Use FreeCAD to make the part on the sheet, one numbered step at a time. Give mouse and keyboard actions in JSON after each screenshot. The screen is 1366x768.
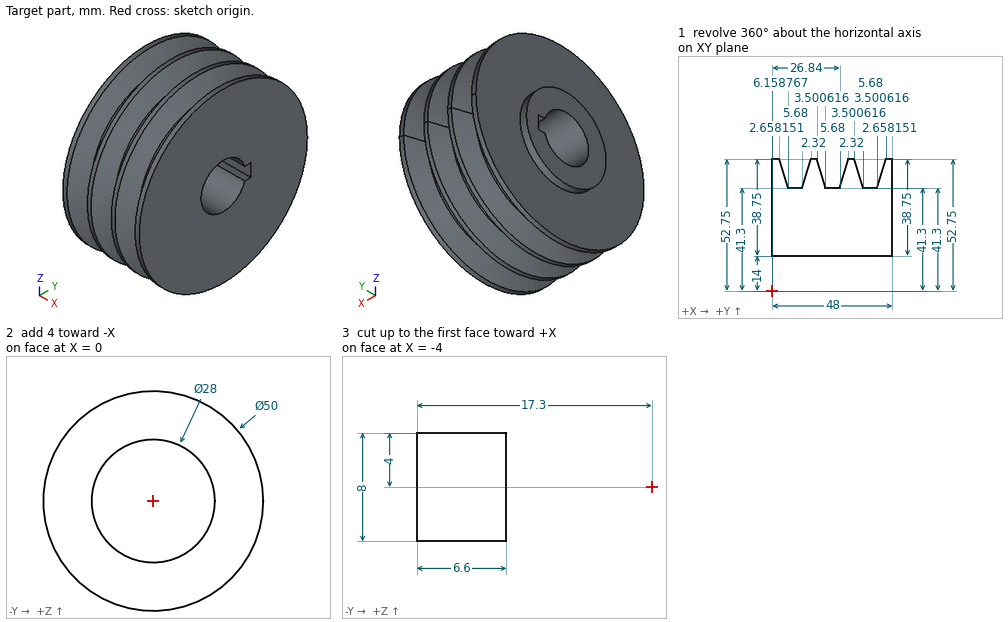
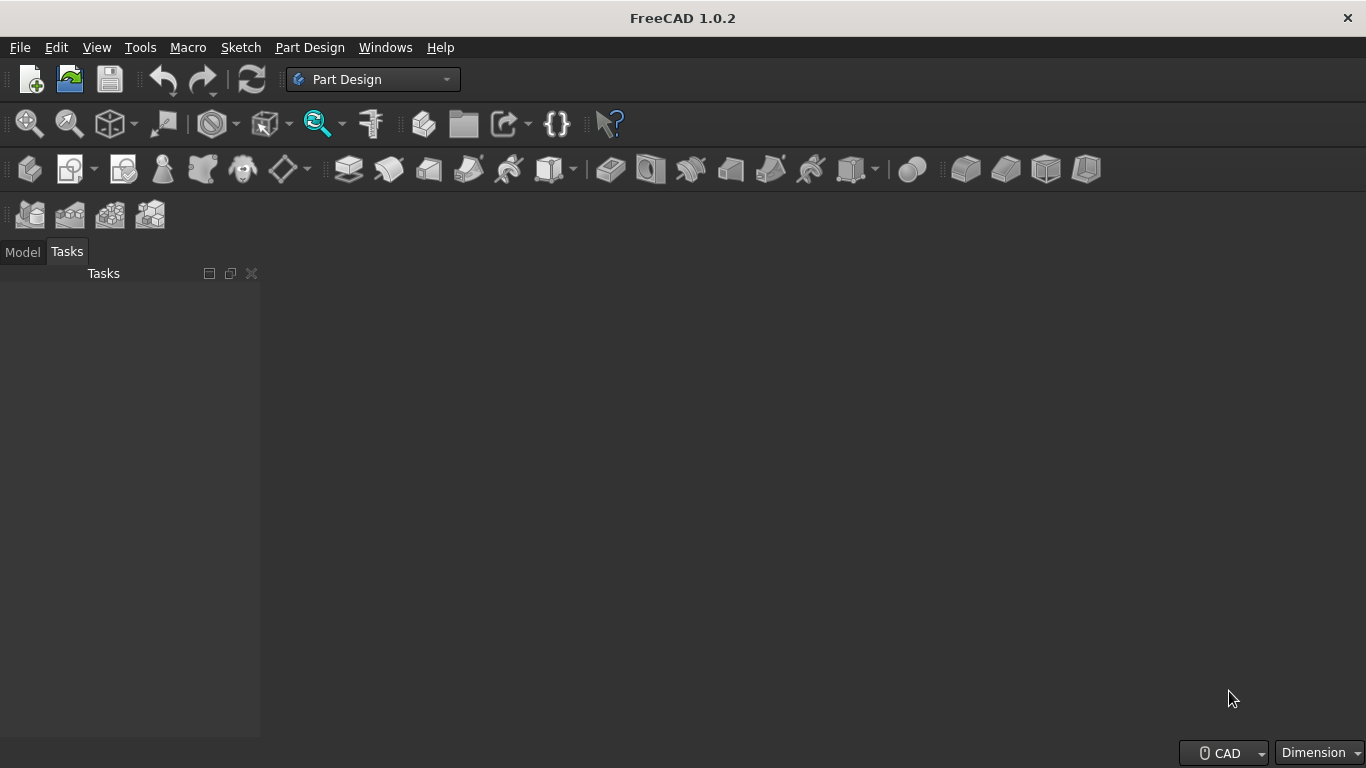
{"action": "left_click", "coordinate": [30, 80]}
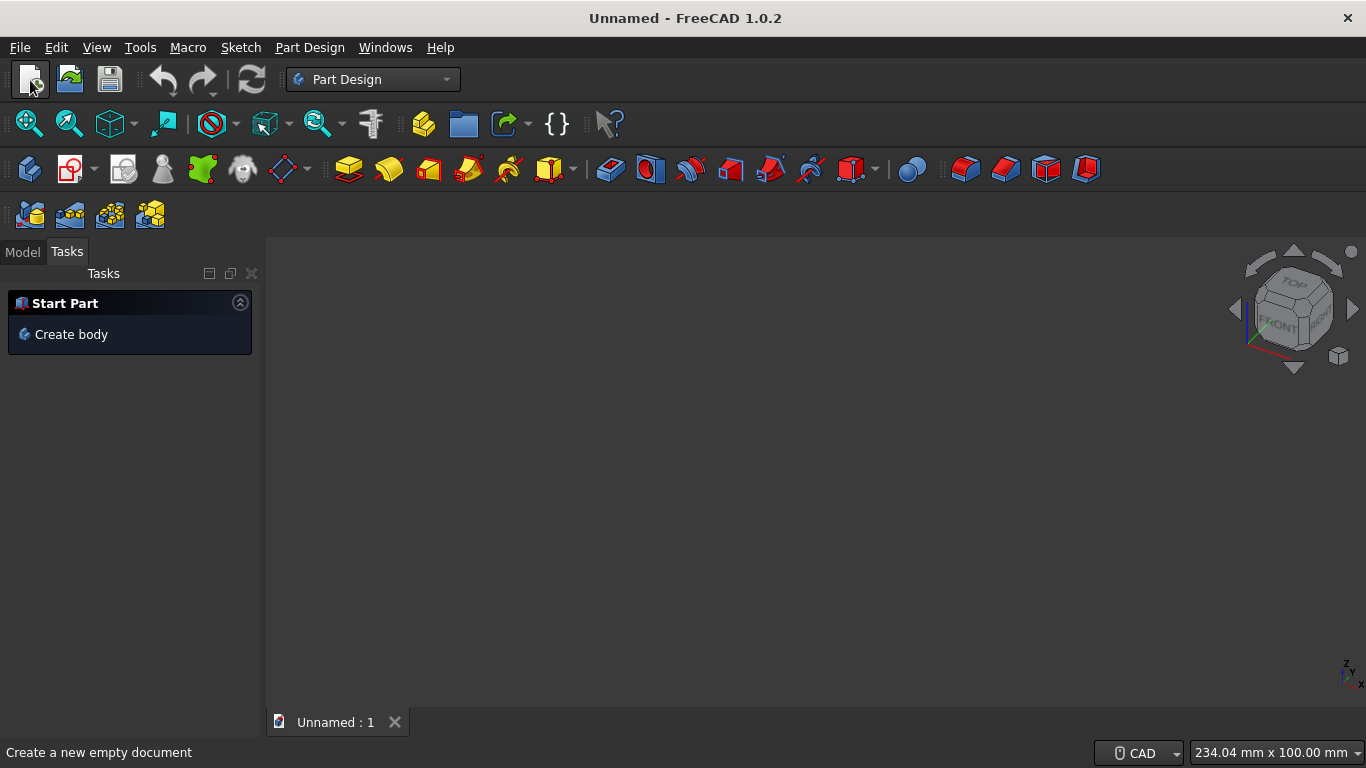
{"action": "left_click", "coordinate": [70, 170]}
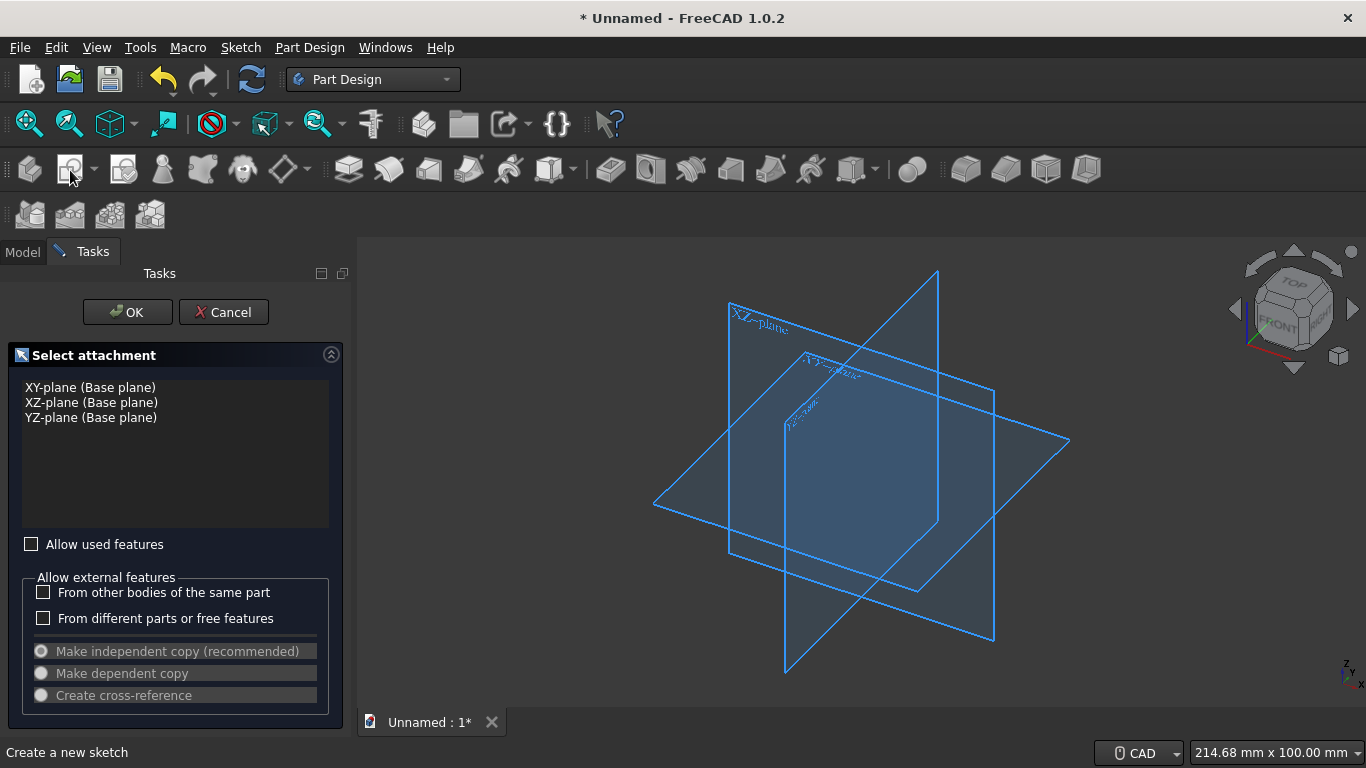
{"action": "left_click", "coordinate": [82, 388]}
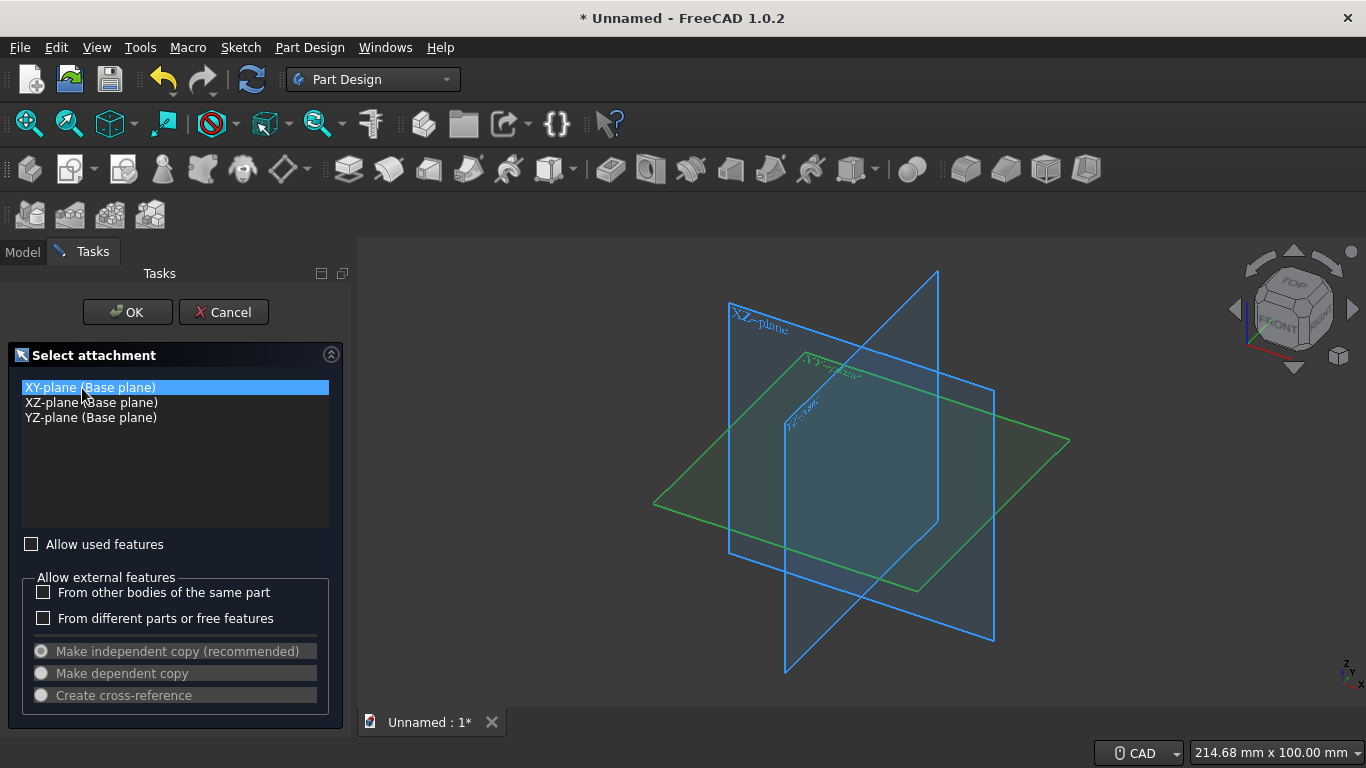
{"action": "left_click", "coordinate": [128, 312]}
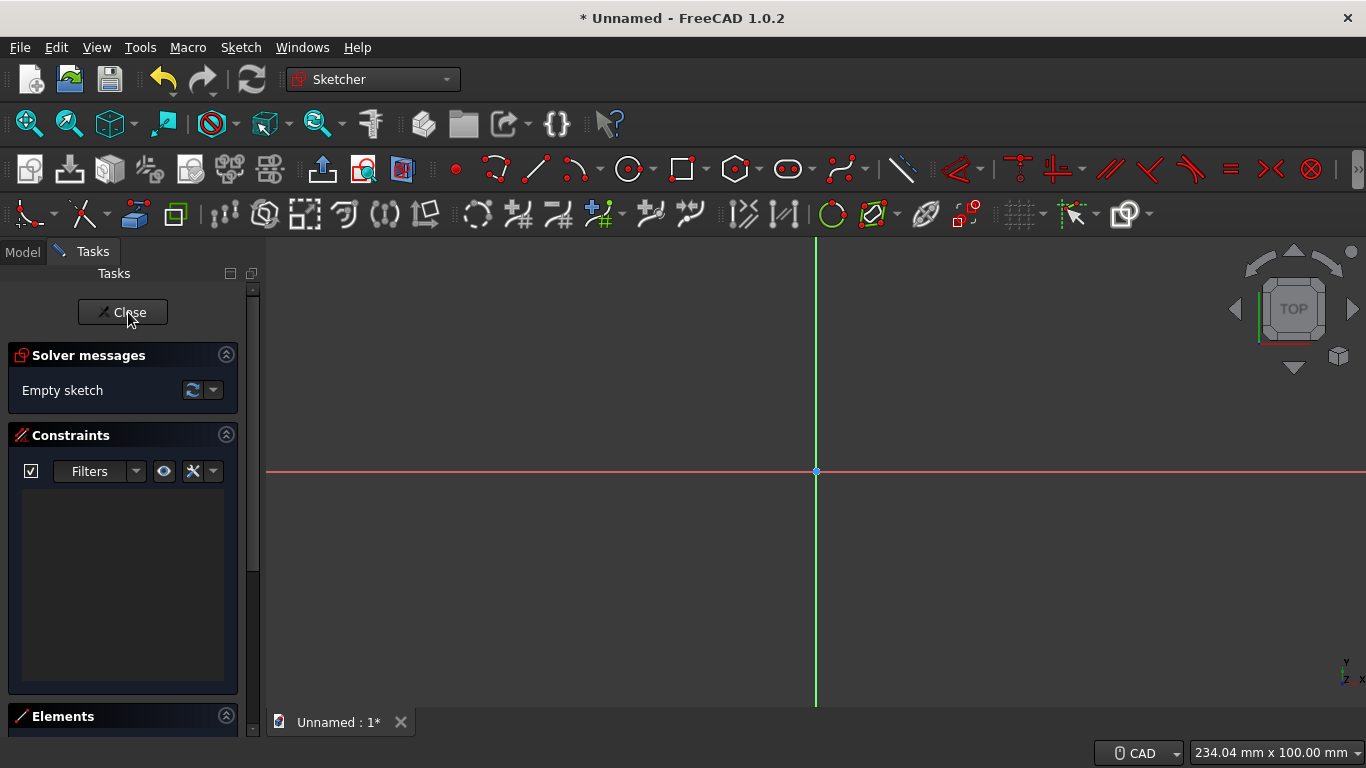
{"action": "scroll", "coordinate": [294, 679], "scroll_direction": "down", "scroll_amount": 1}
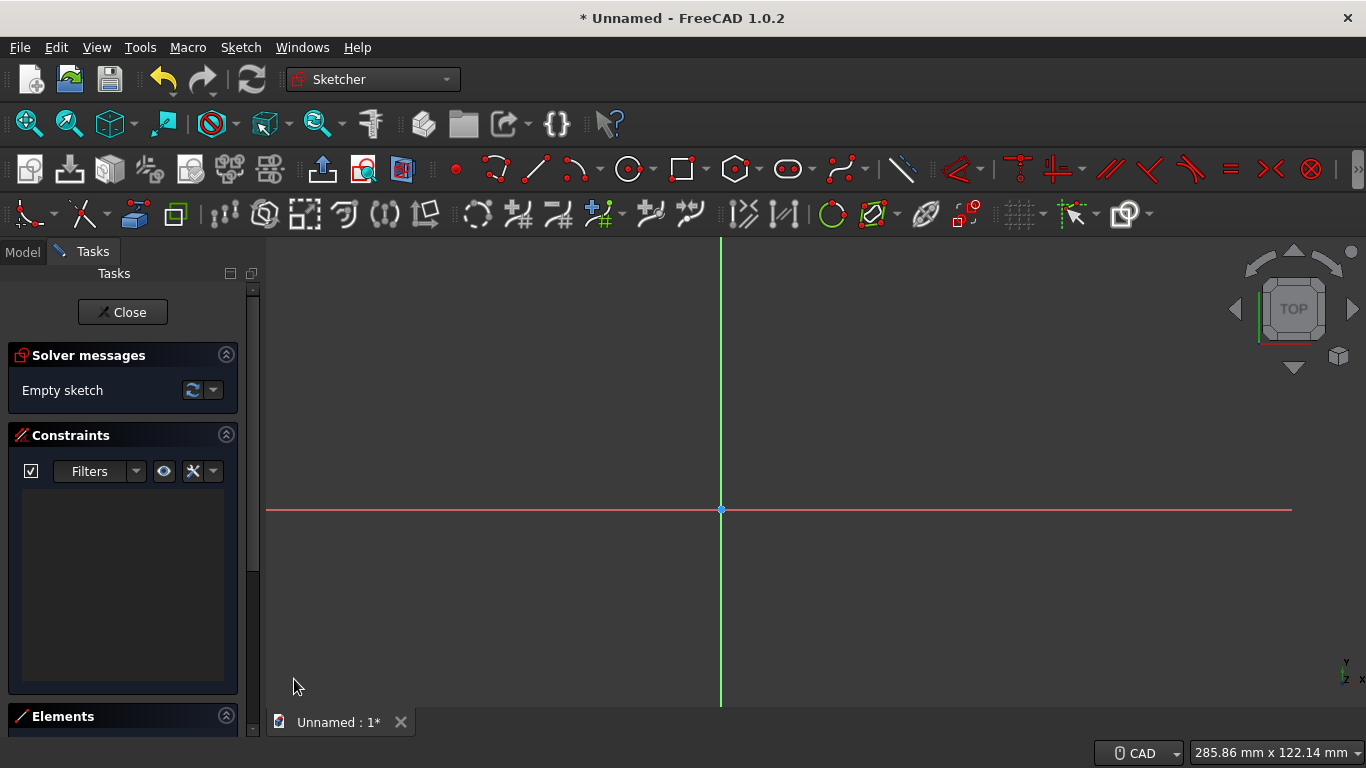
{"action": "scroll", "coordinate": [948, 278], "scroll_direction": "up", "scroll_amount": 2}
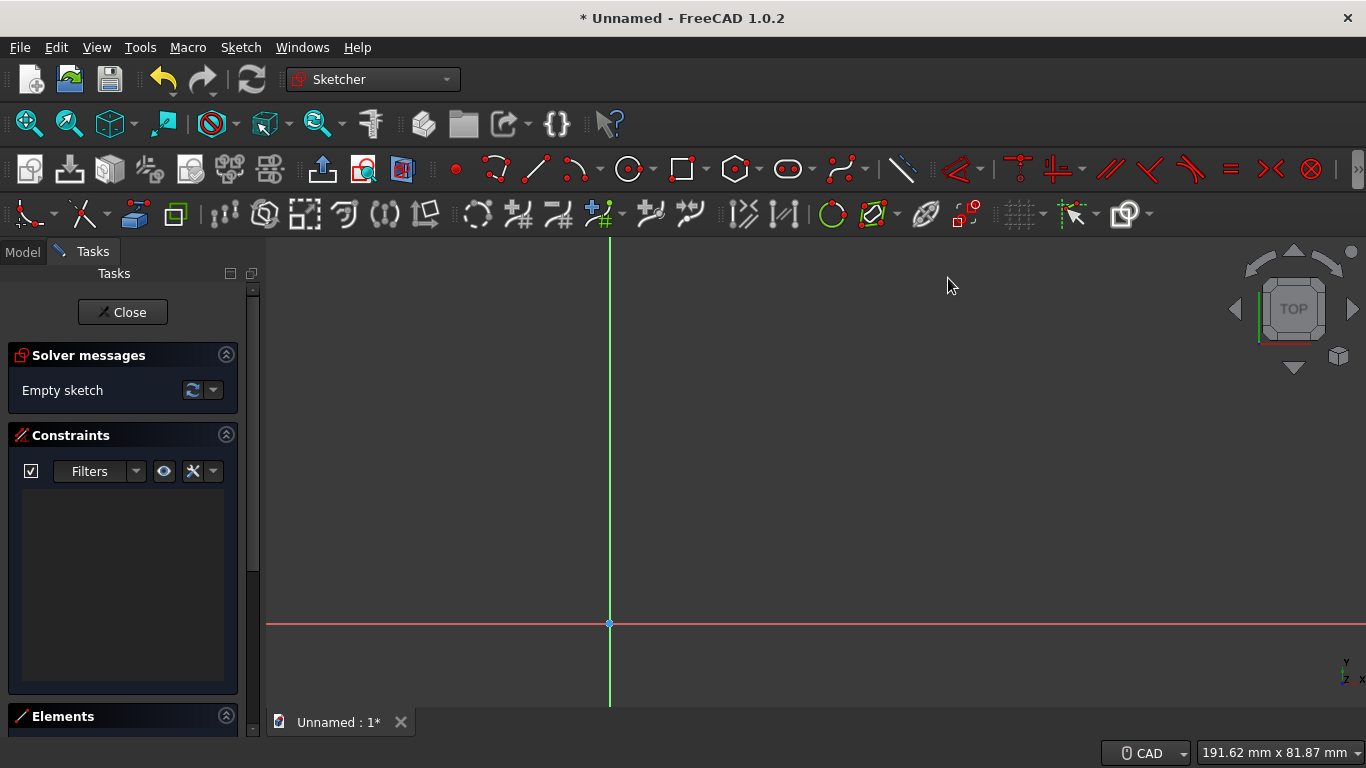
{"action": "left_click", "coordinate": [496, 170]}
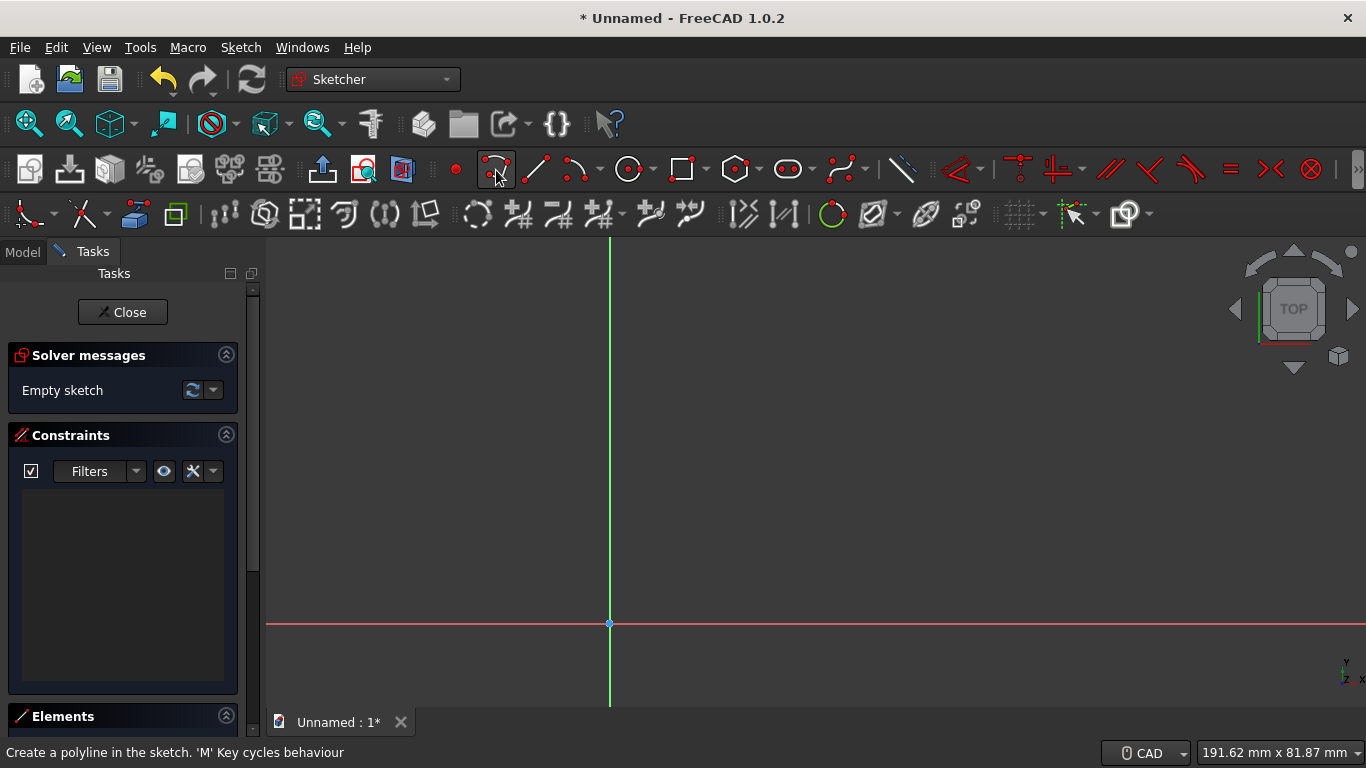
{"action": "left_click", "coordinate": [610, 543]}
{"action": "left_click", "coordinate": [885, 543]}
{"action": "left_click", "coordinate": [885, 321]}
{"action": "left_click", "coordinate": [870, 321]}
{"action": "left_click", "coordinate": [850, 387]}
{"action": "left_click", "coordinate": [817, 387]}
{"action": "left_click", "coordinate": [797, 321]}
{"action": "left_click", "coordinate": [784, 321]}
{"action": "left_click", "coordinate": [764, 387]}
{"action": "left_click", "coordinate": [731, 387]}
{"action": "left_click", "coordinate": [711, 321]}
{"action": "left_click", "coordinate": [698, 321]}
{"action": "left_click", "coordinate": [678, 387]}
{"action": "left_click", "coordinate": [645, 387]}
{"action": "left_click", "coordinate": [625, 321]}
{"action": "left_click", "coordinate": [619, 321]}
{"action": "left_click", "coordinate": [610, 544]}
{"action": "key", "text": "Escape"}
{"action": "key", "text": "Escape"}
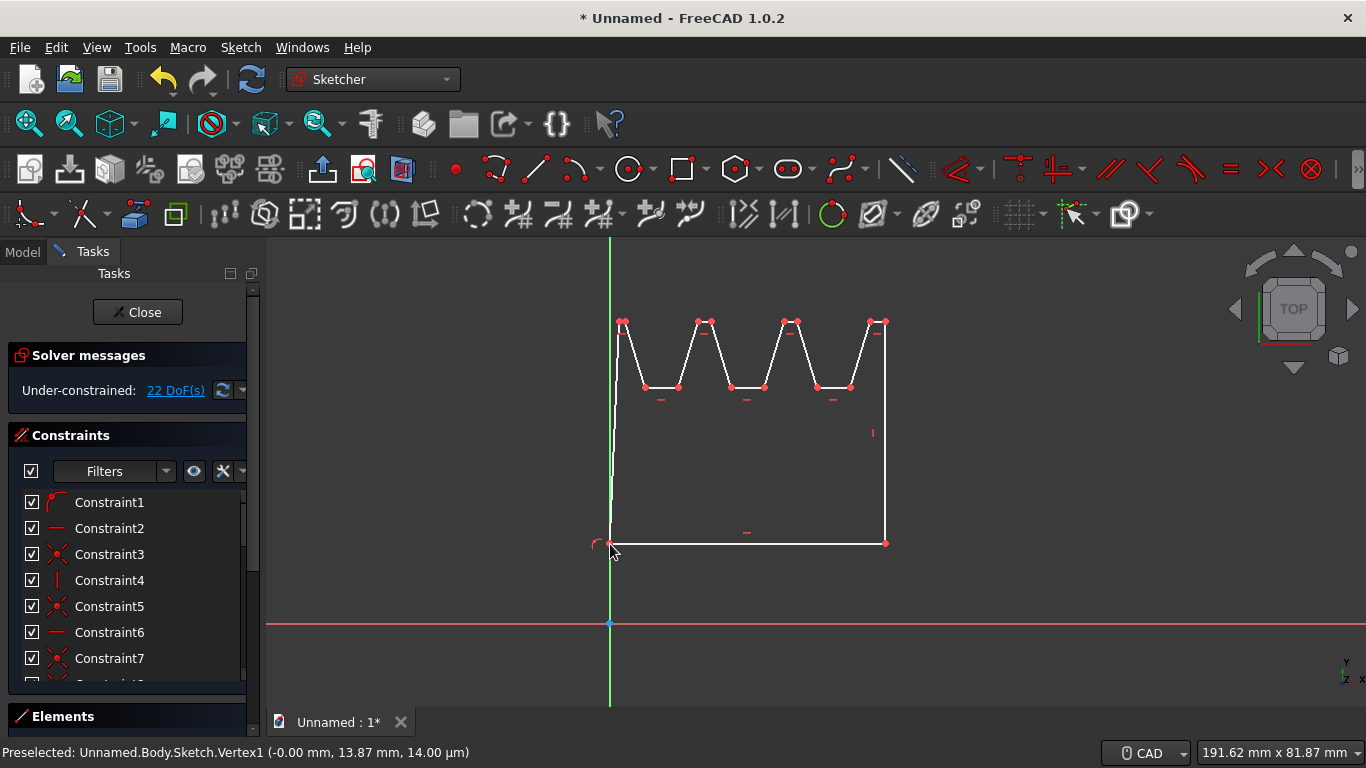
{"action": "left_click", "coordinate": [612, 477]}